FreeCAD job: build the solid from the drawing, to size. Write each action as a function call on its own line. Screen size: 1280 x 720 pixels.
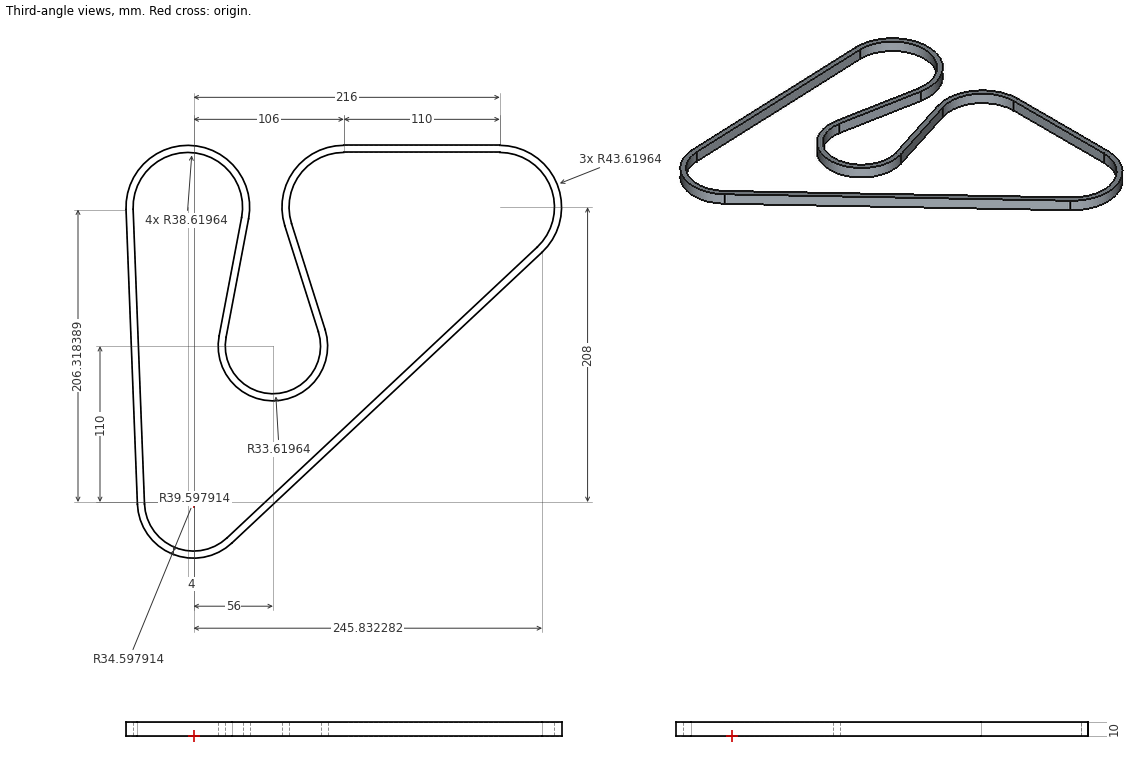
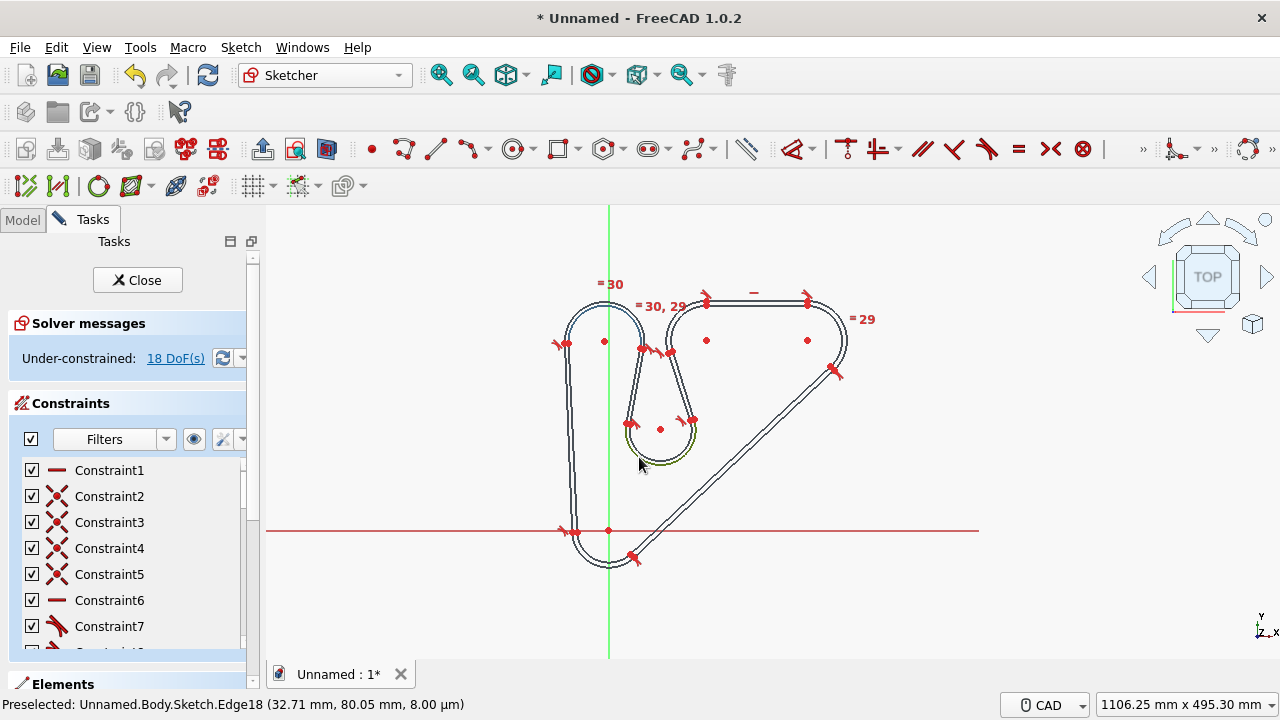
scroll(688, 311, up, 6)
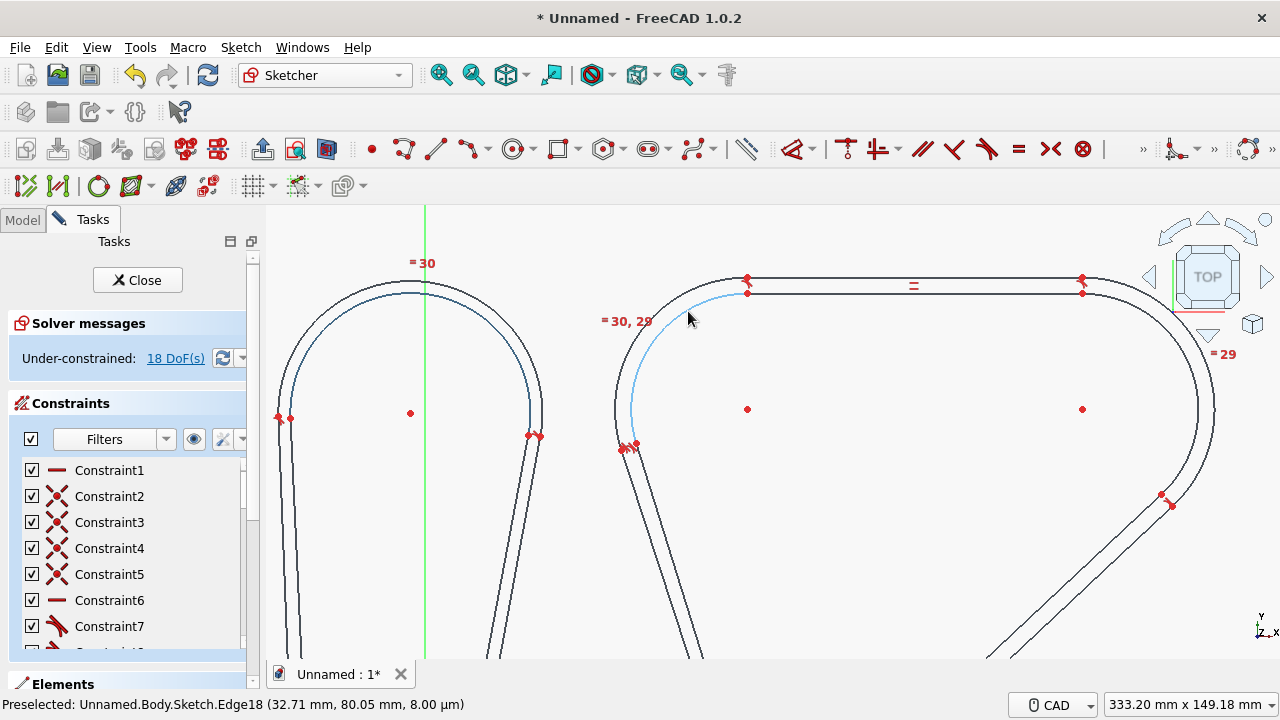
click(685, 312)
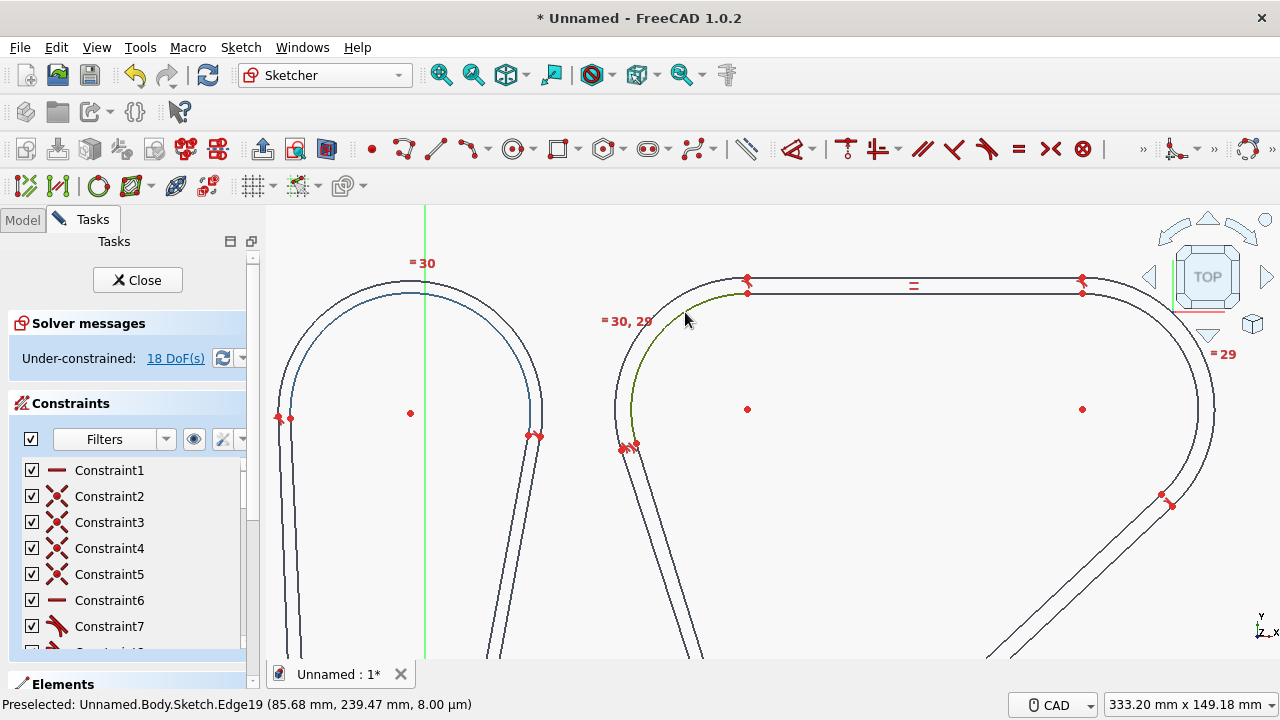
click(1020, 150)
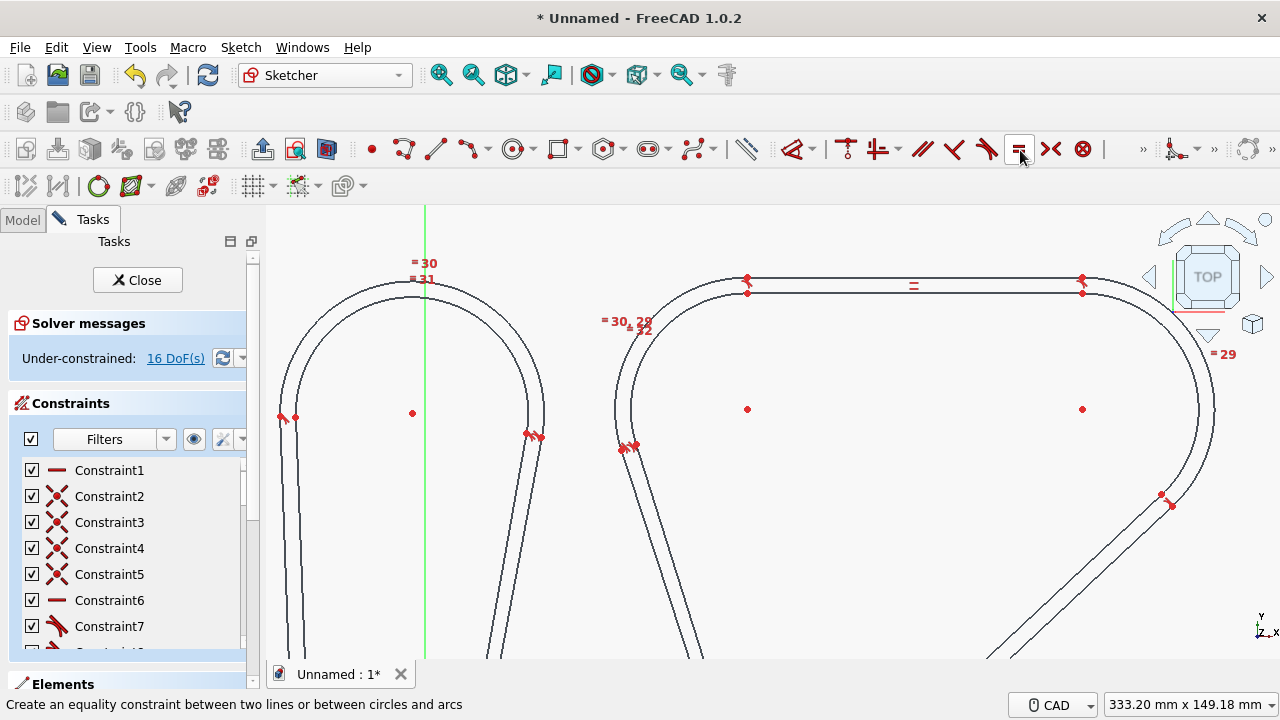
scroll(688, 311, down, 6)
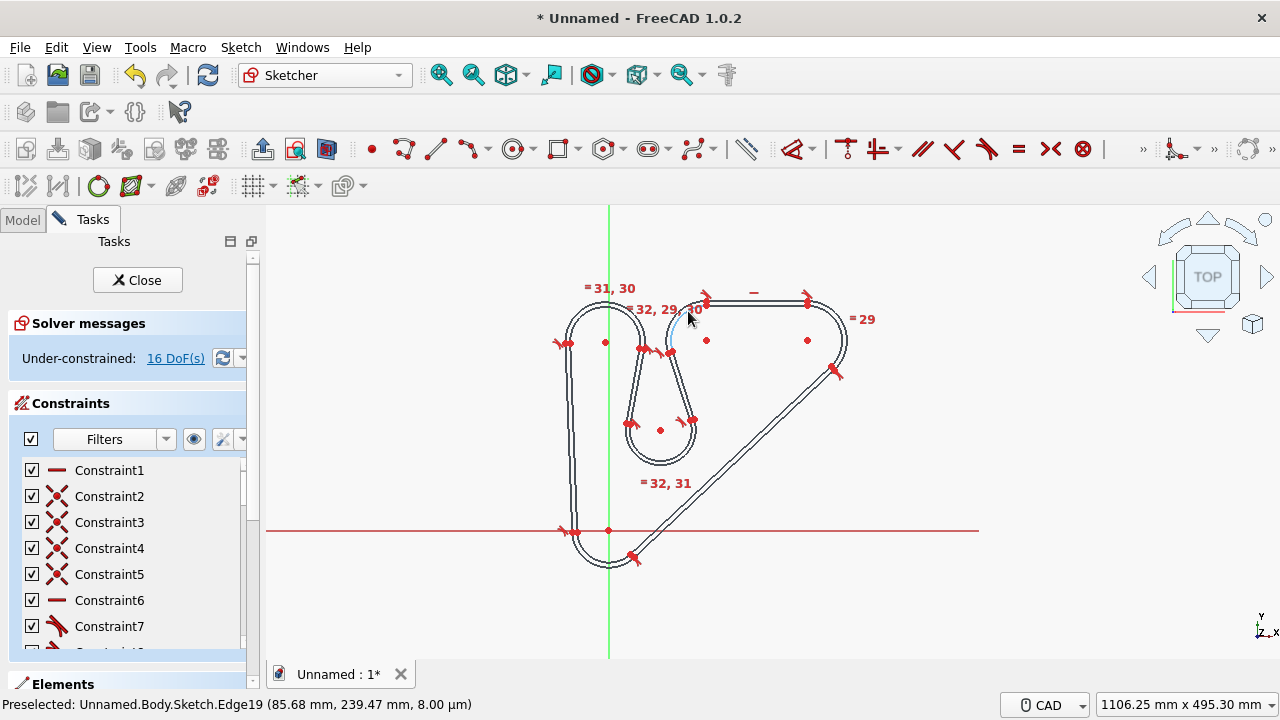
scroll(847, 345, up, 6)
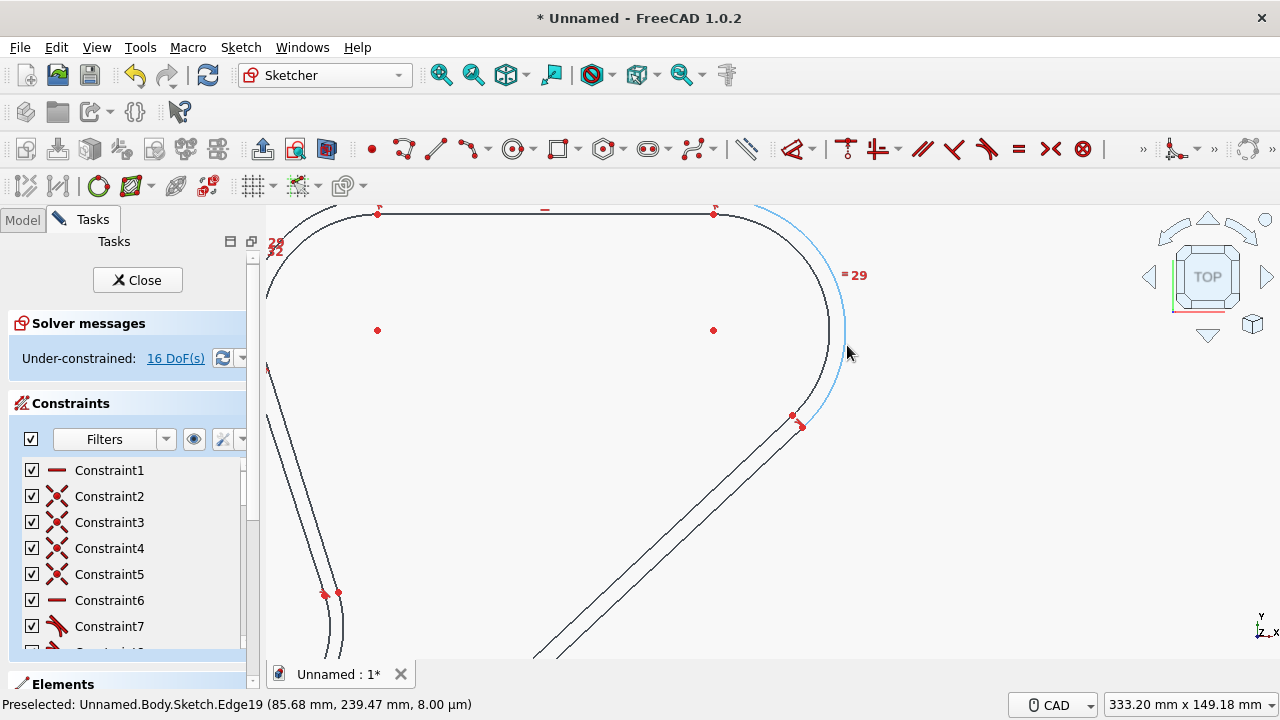
click(845, 344)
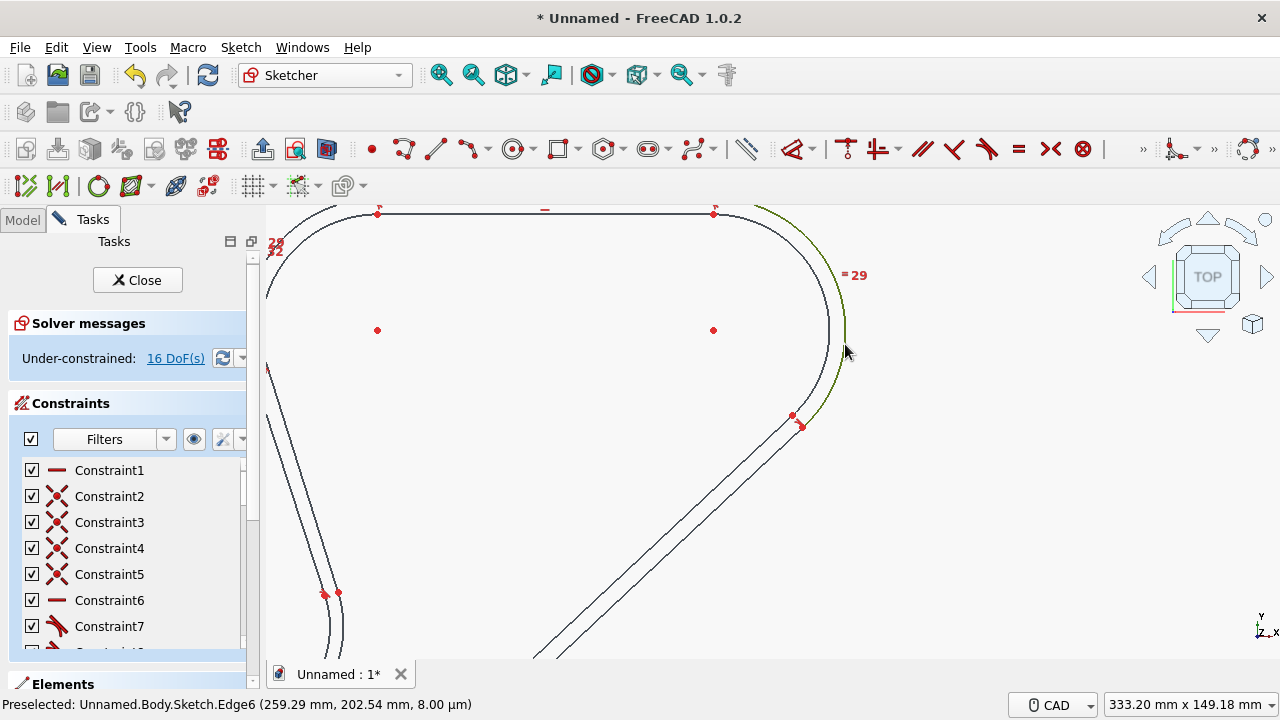
key(k)
key(r)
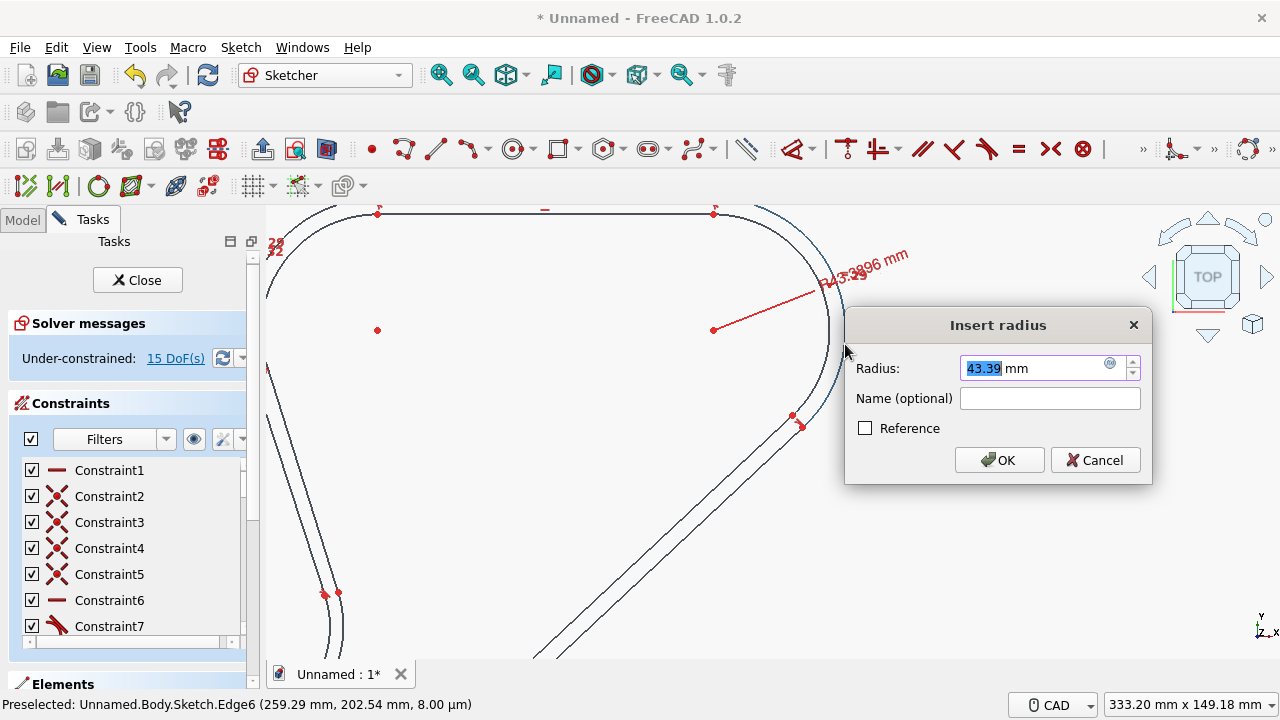
text(43.61964)
key(Return)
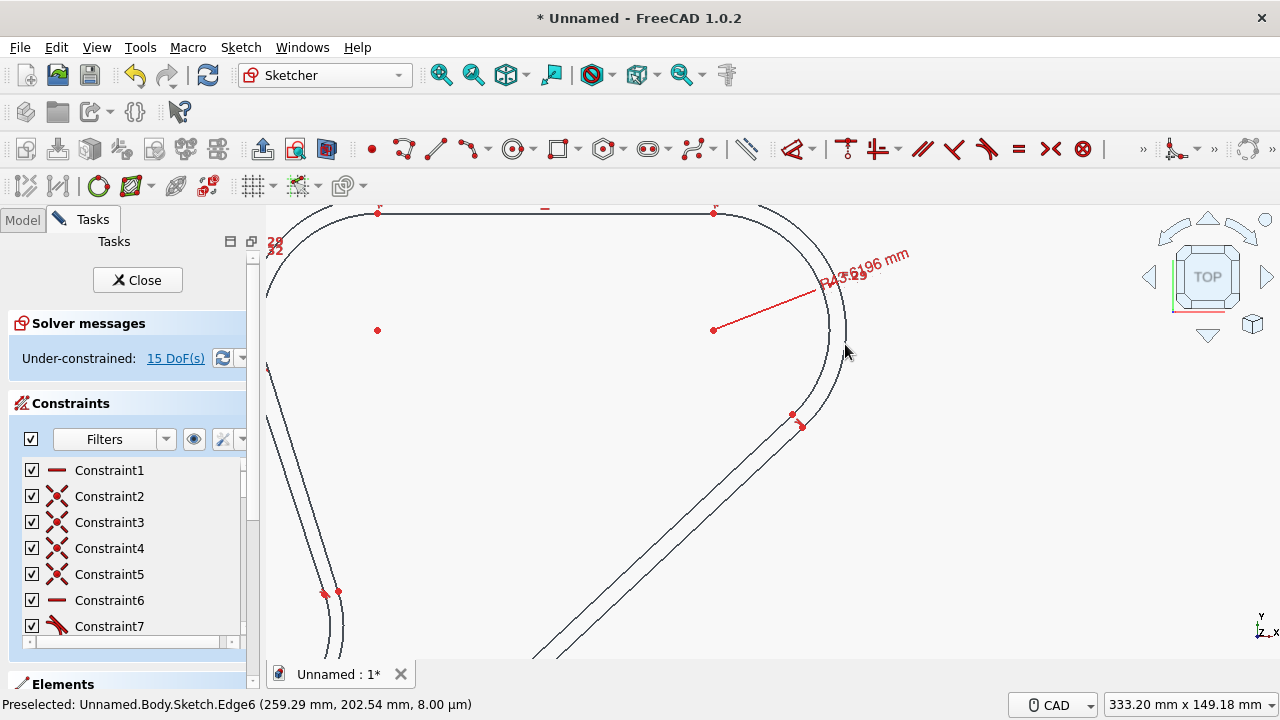
scroll(847, 345, down, 6)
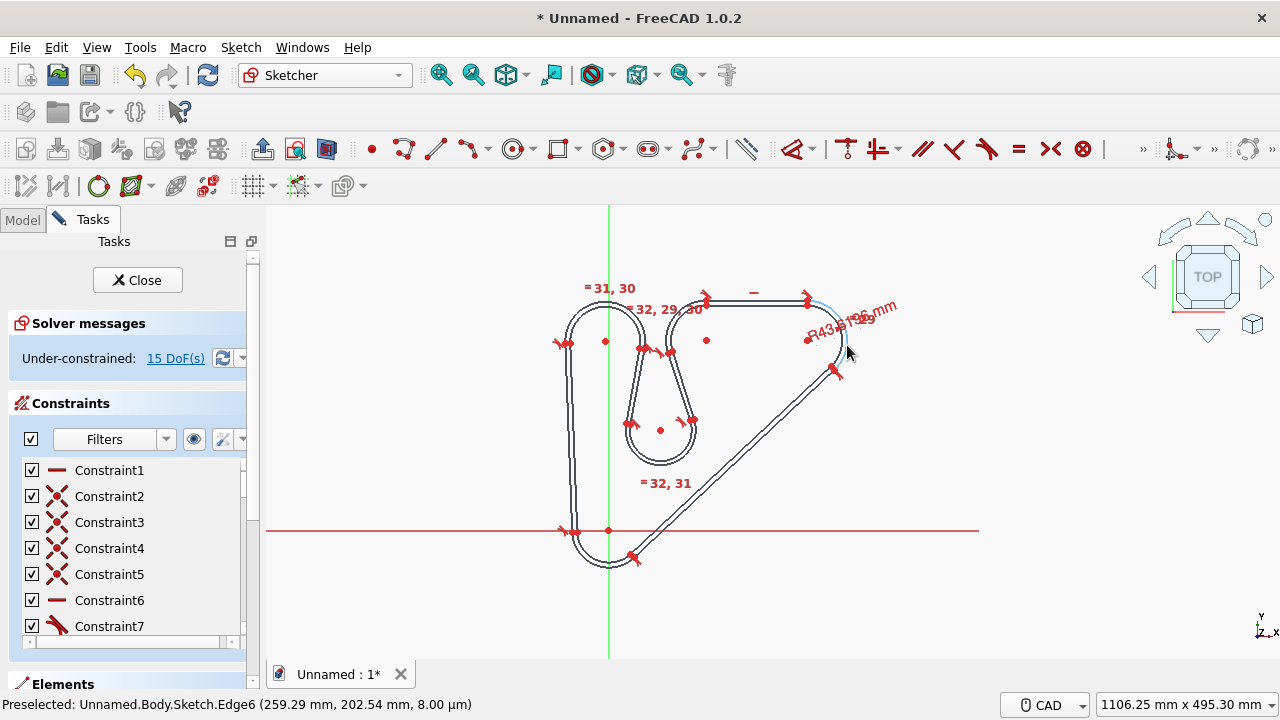
scroll(642, 454, up, 7)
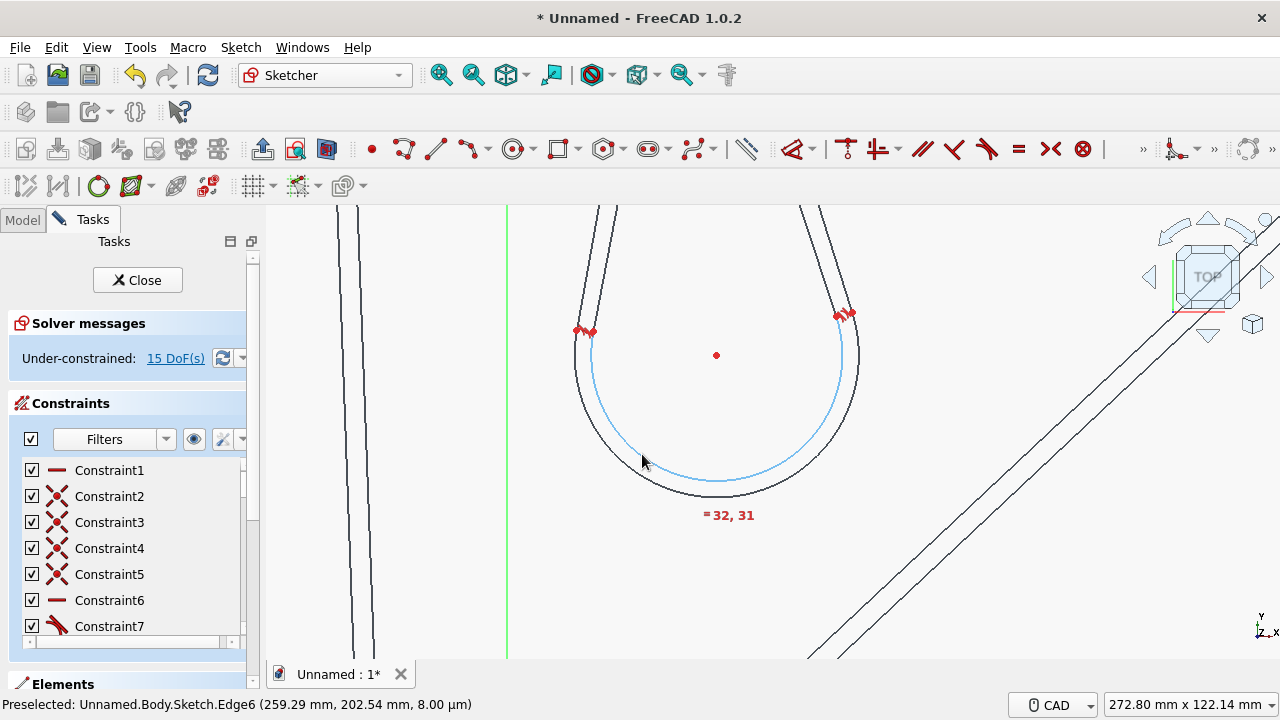
click(639, 454)